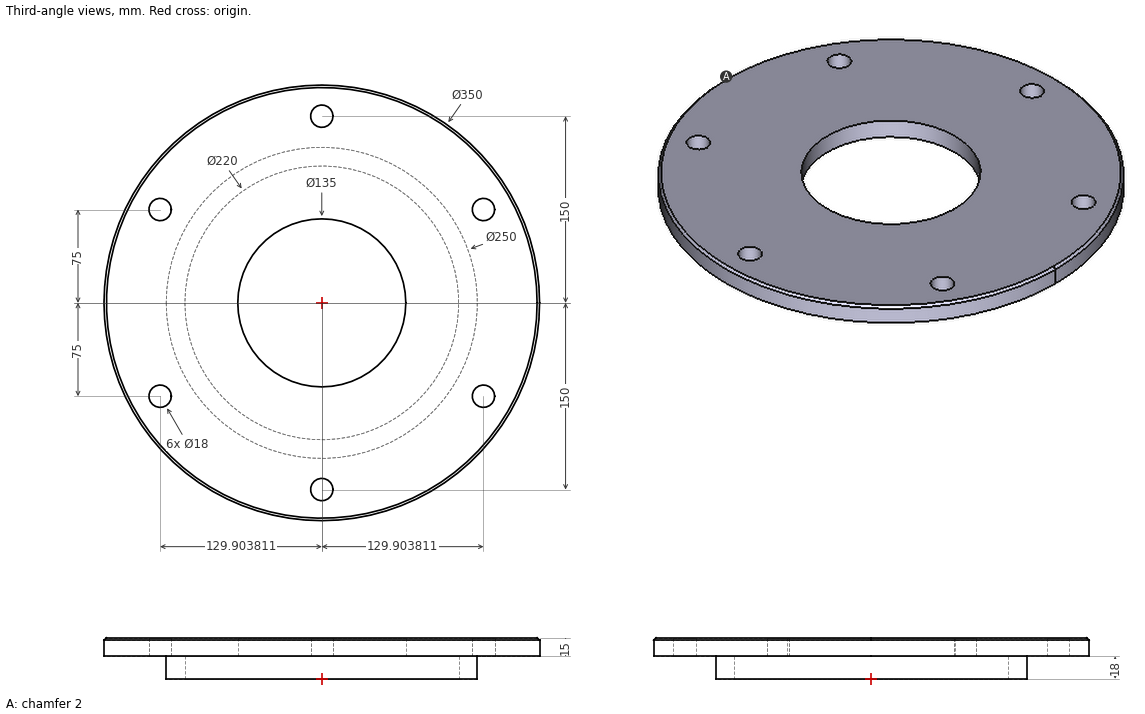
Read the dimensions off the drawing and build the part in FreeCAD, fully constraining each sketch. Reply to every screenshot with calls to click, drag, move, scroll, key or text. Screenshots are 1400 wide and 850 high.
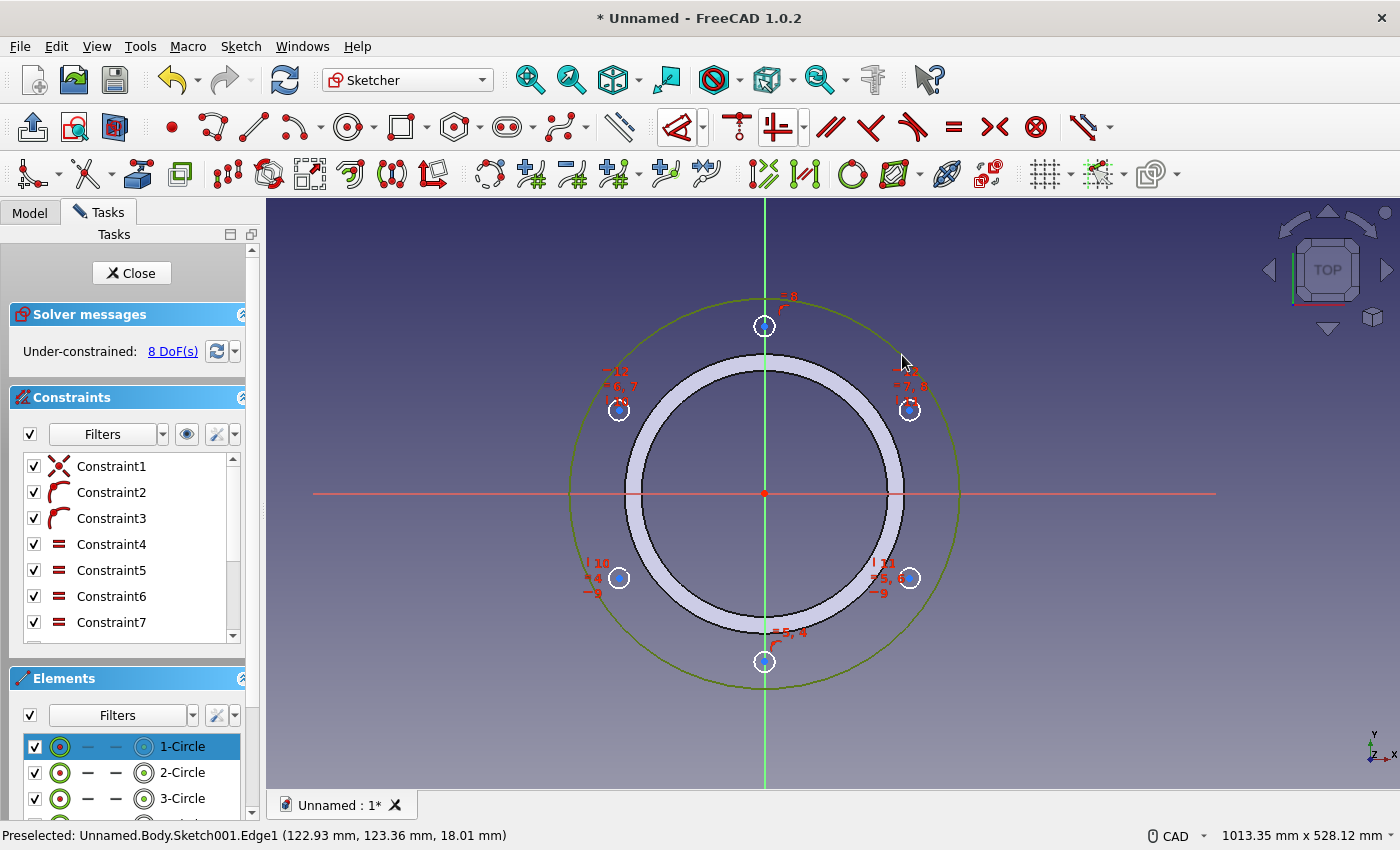
key(k)
key(o)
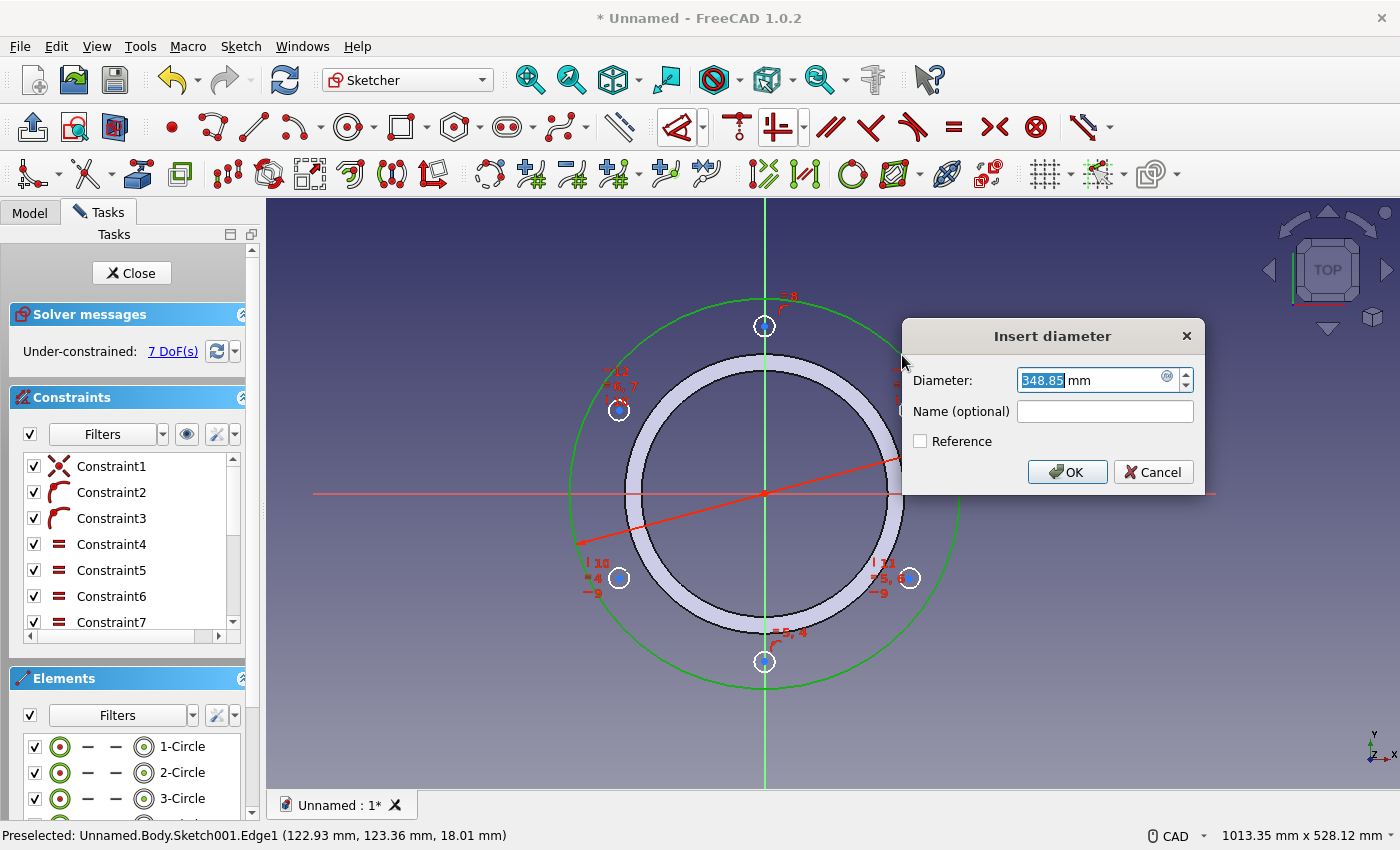
text(350)
key(Return)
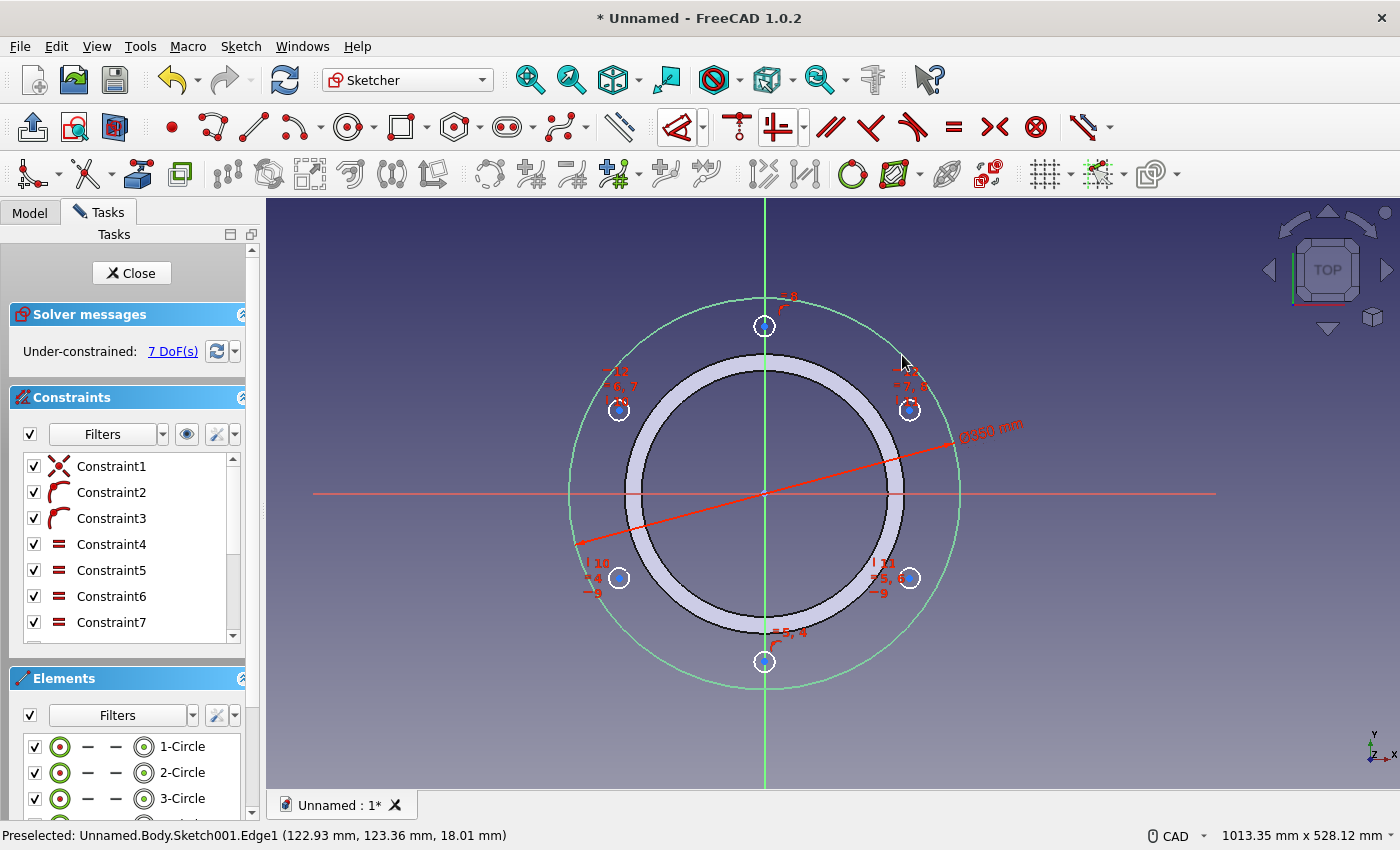
scroll(626, 571, up, 4)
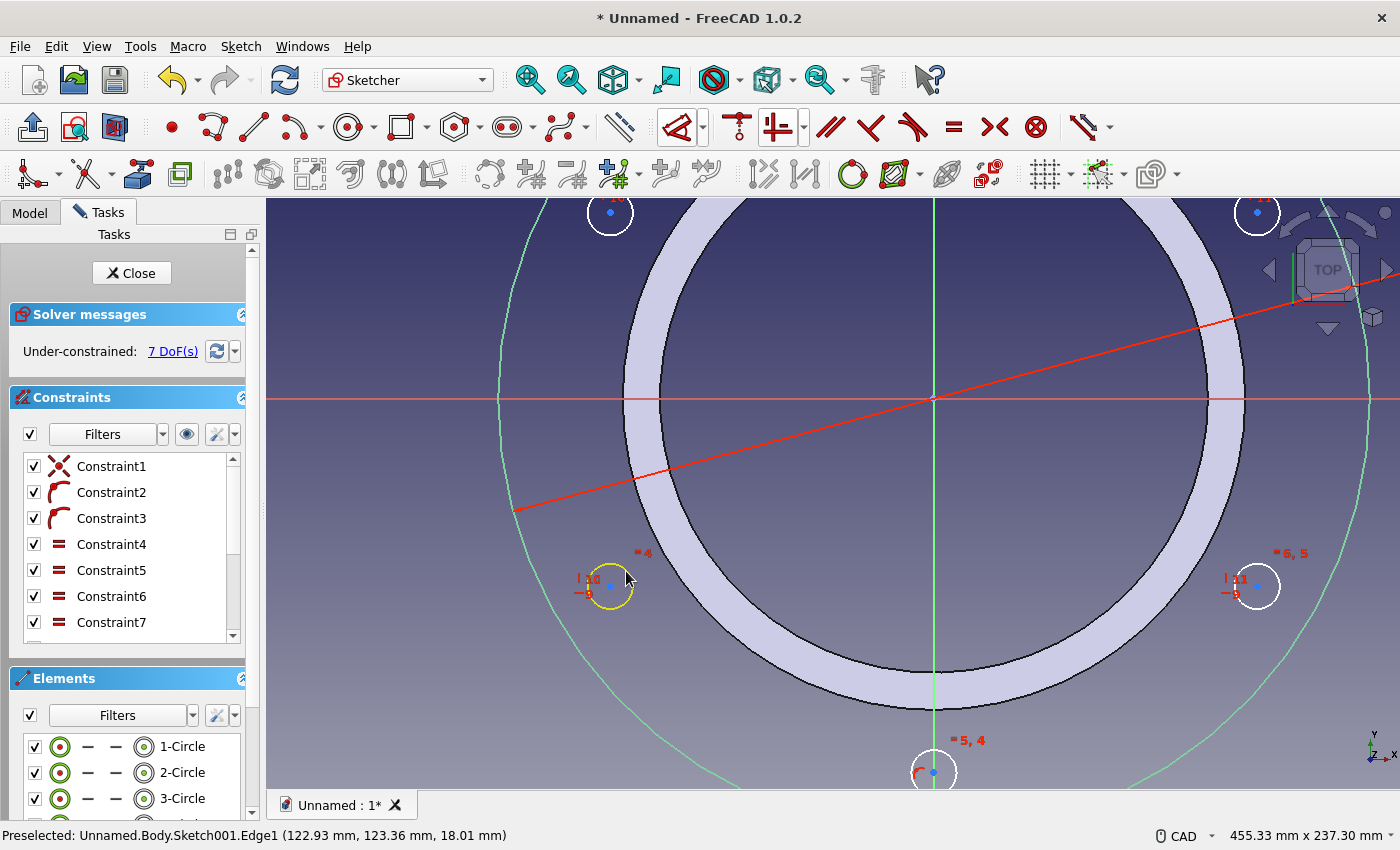
click(626, 570)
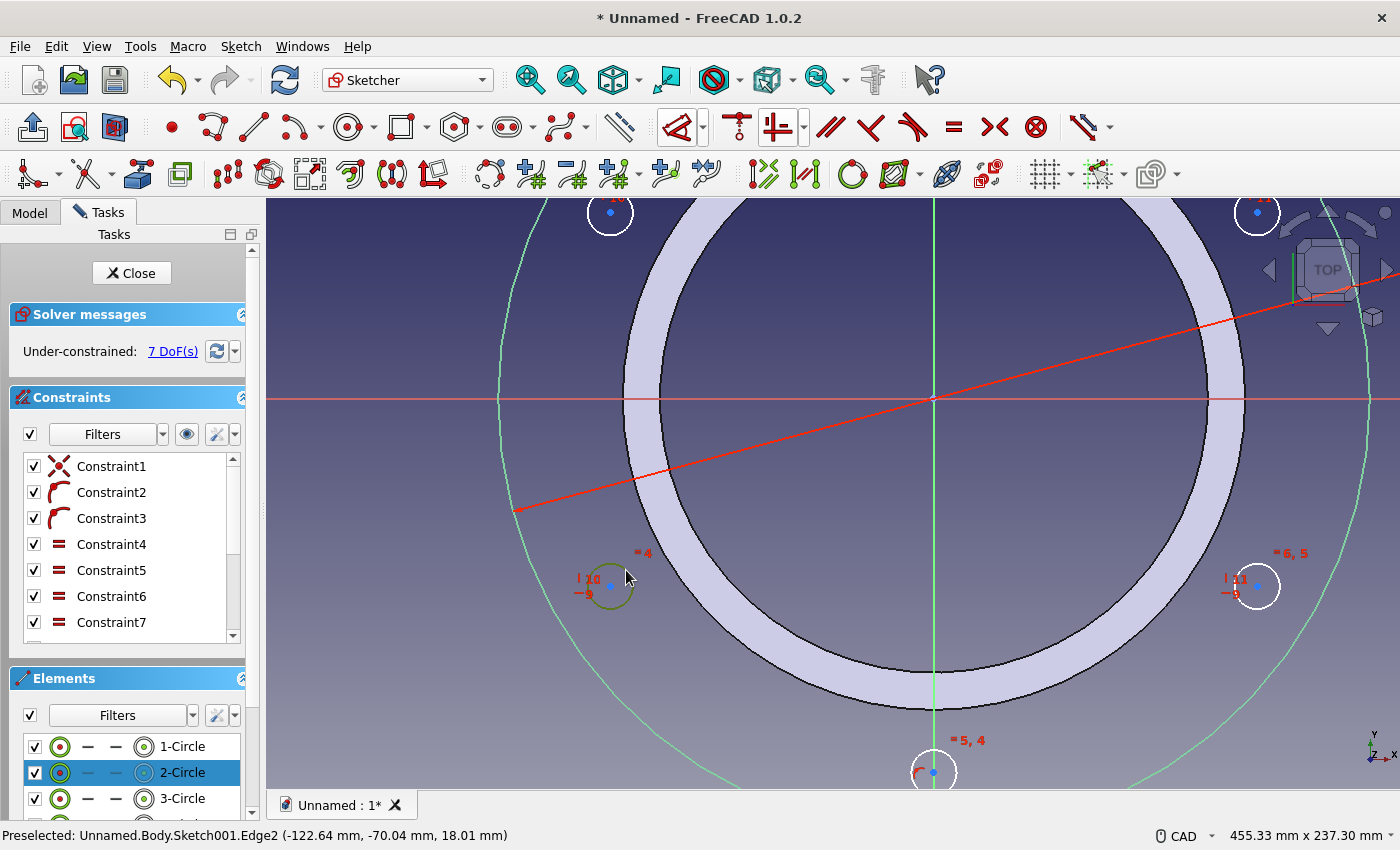
key(k)
key(o)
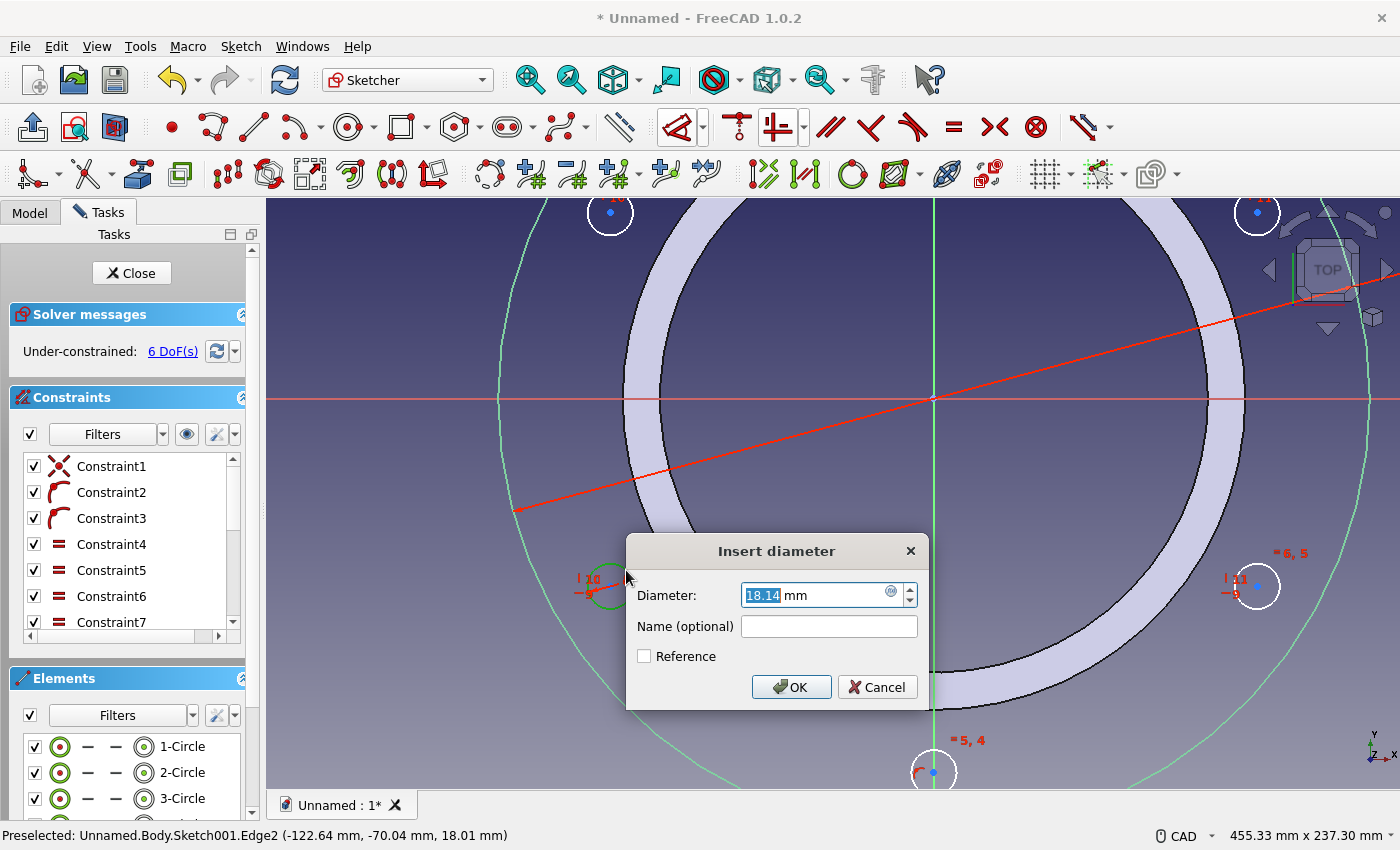
text(18)
key(Return)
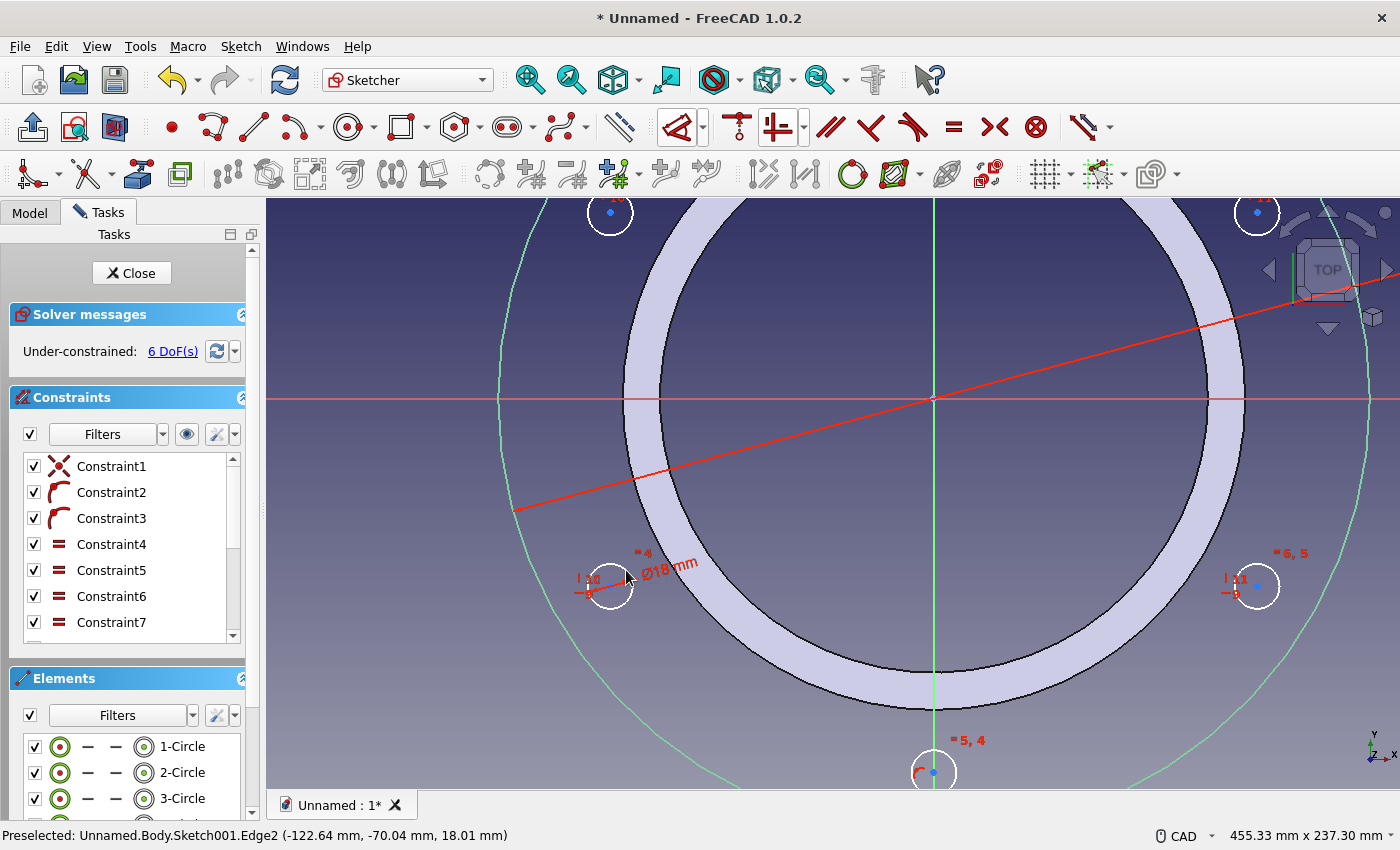
click(610, 586)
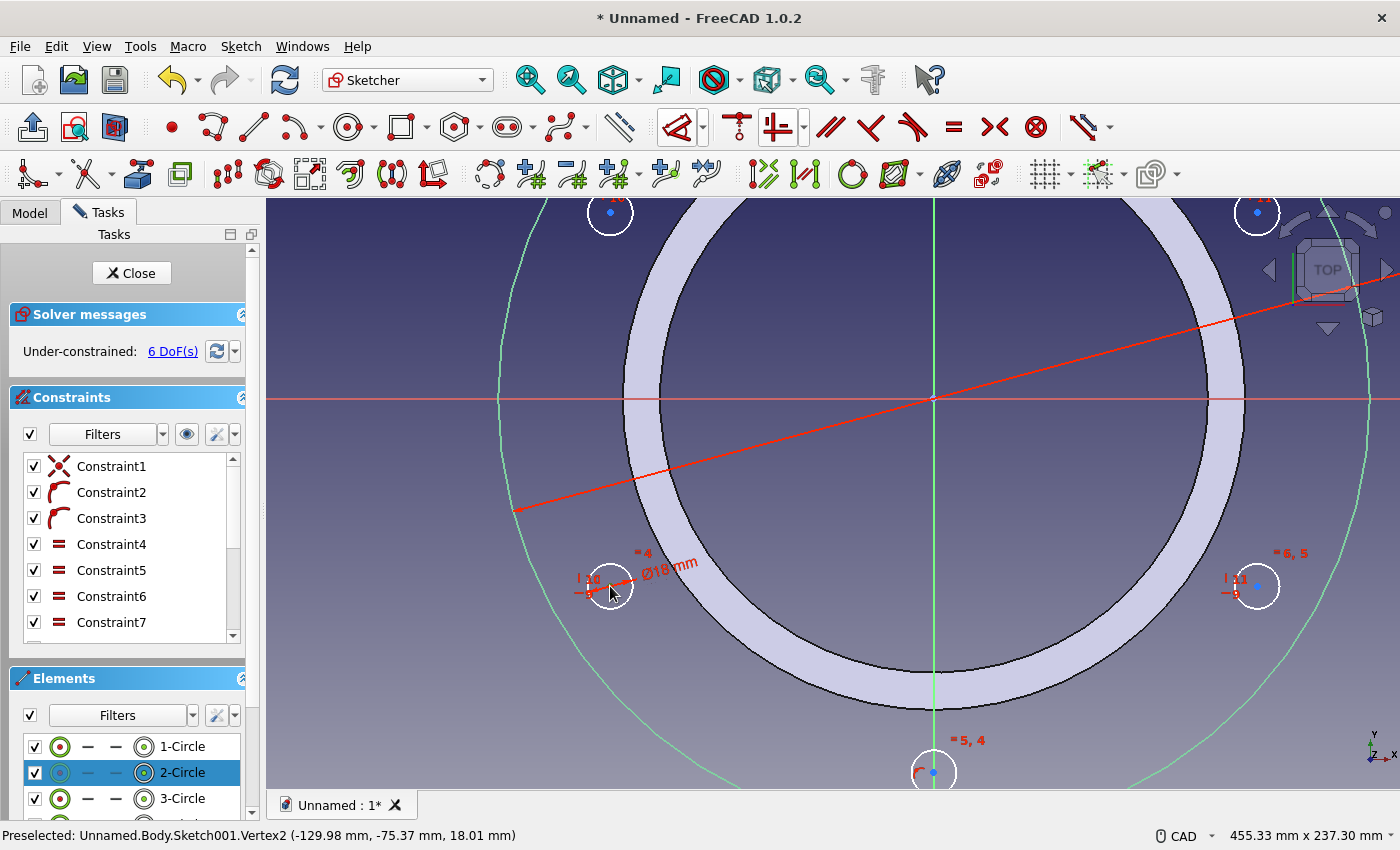
key(i)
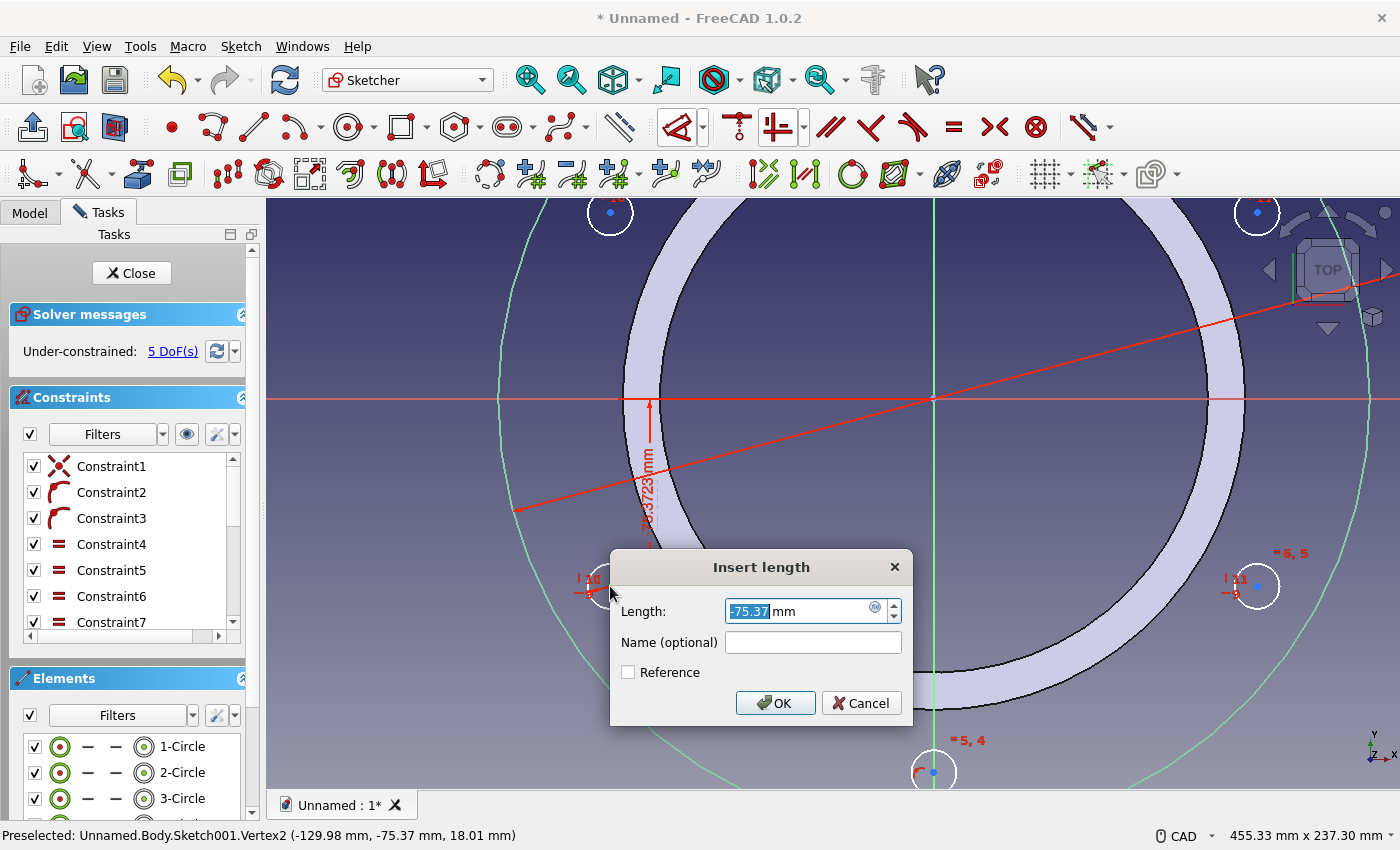
text(-75)
key(Return)